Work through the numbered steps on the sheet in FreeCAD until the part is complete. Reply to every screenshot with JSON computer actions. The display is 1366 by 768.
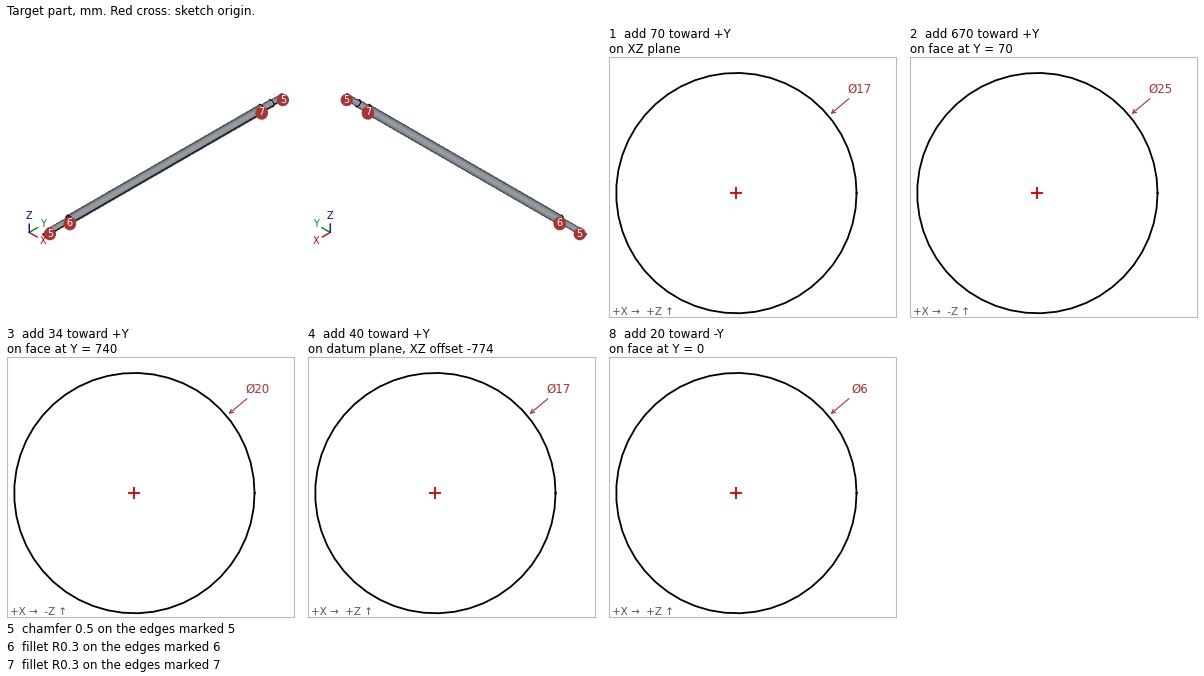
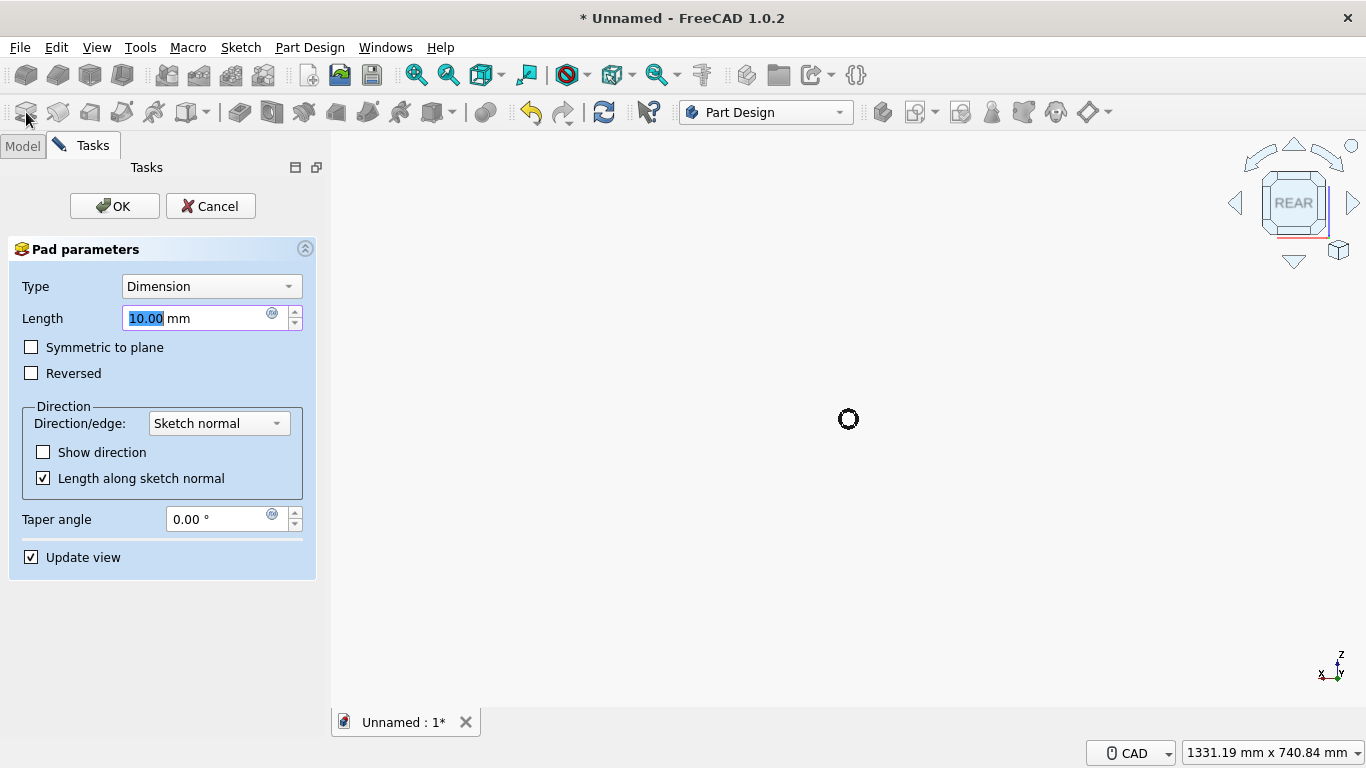
{"action": "type", "text": "34"}
{"action": "key", "text": "Tab"}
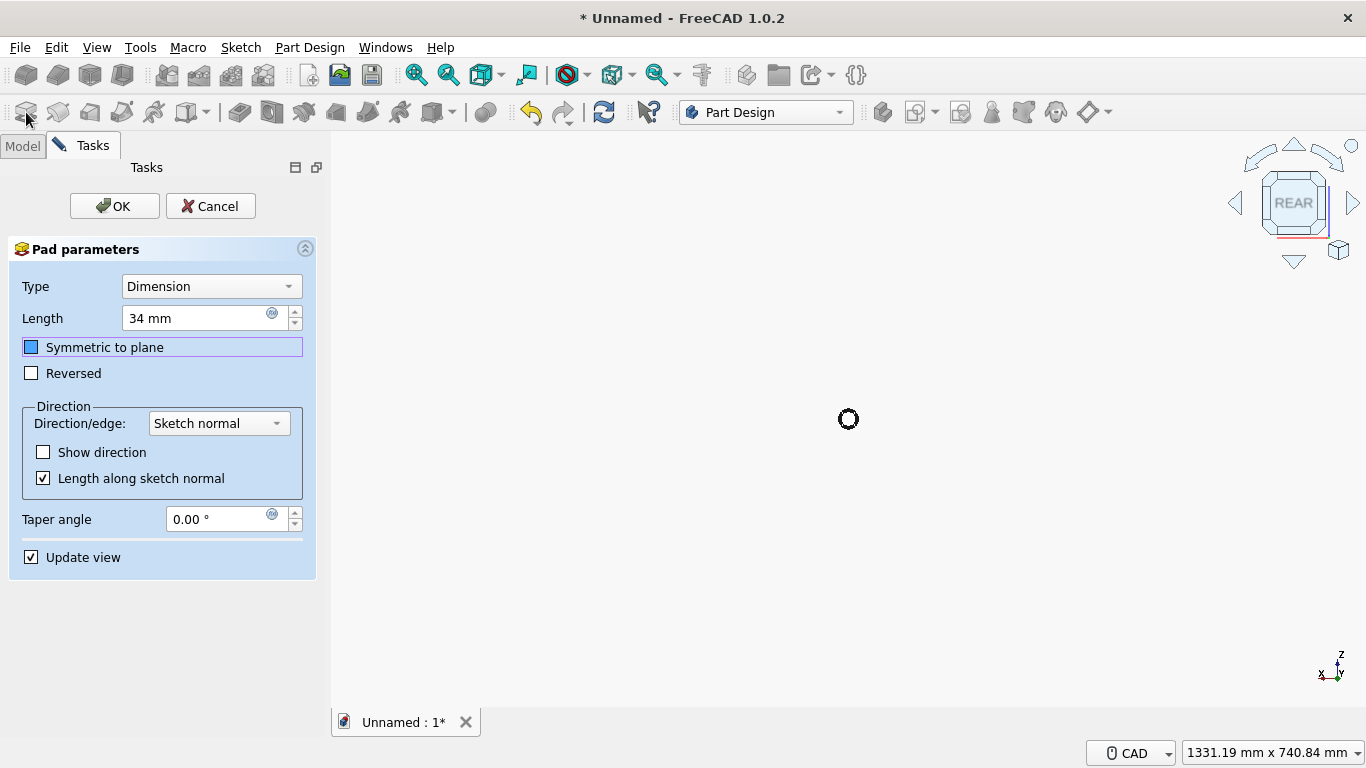
{"action": "left_click", "coordinate": [115, 206]}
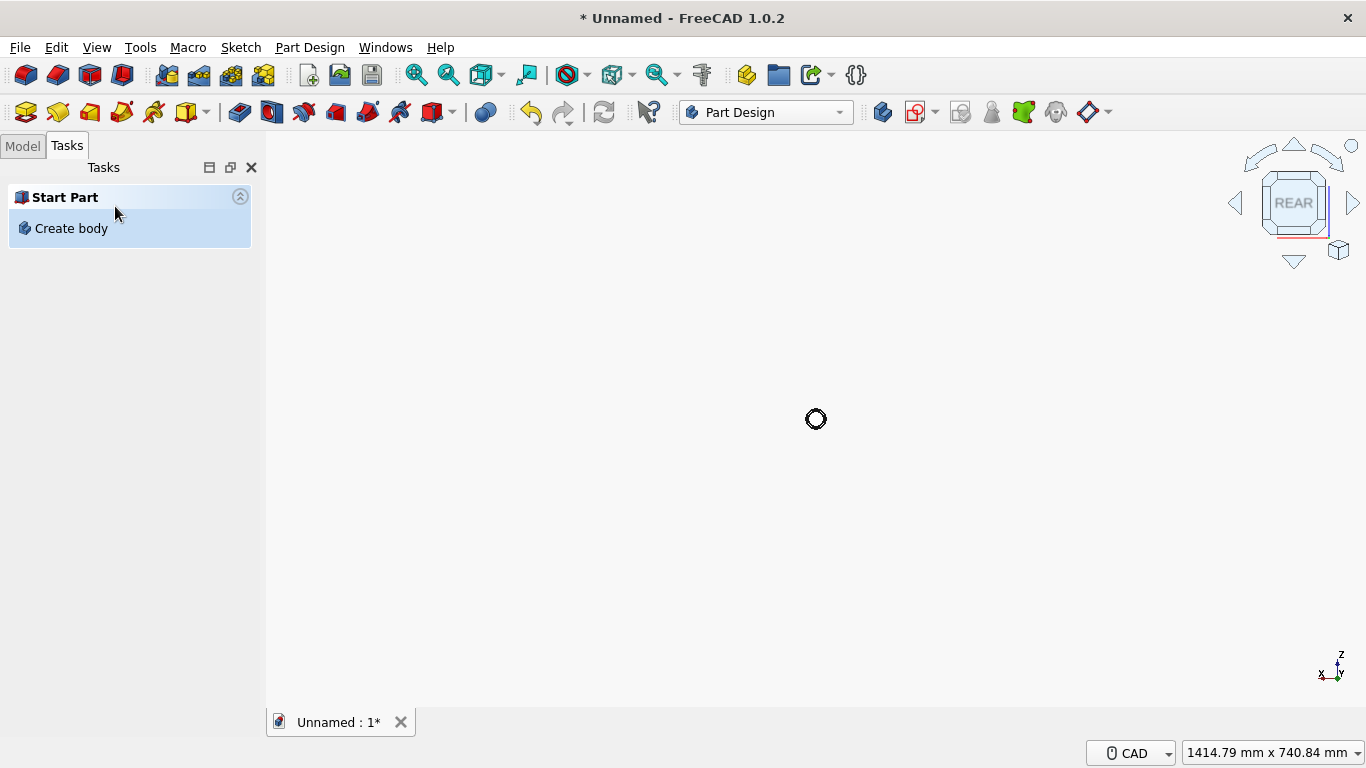
{"action": "left_click", "coordinate": [418, 76]}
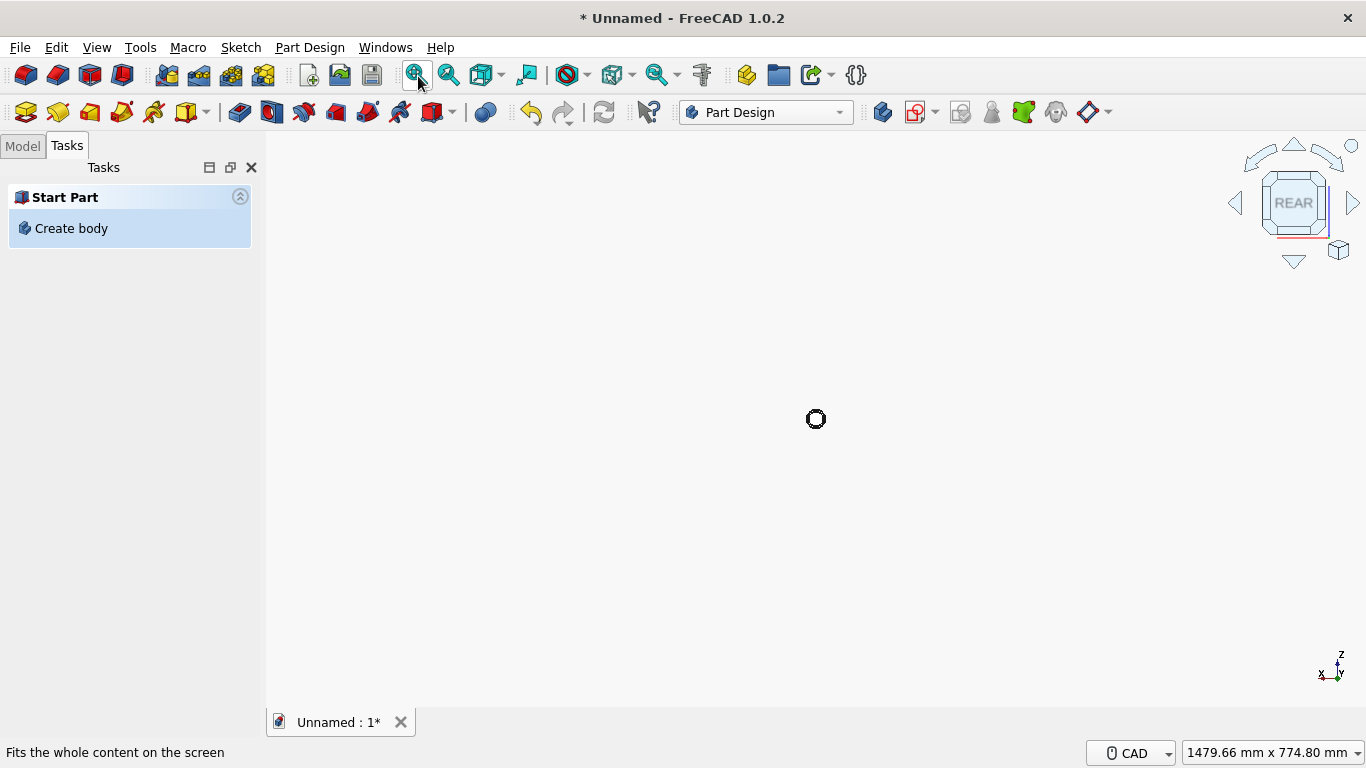
{"action": "key", "text": "5"}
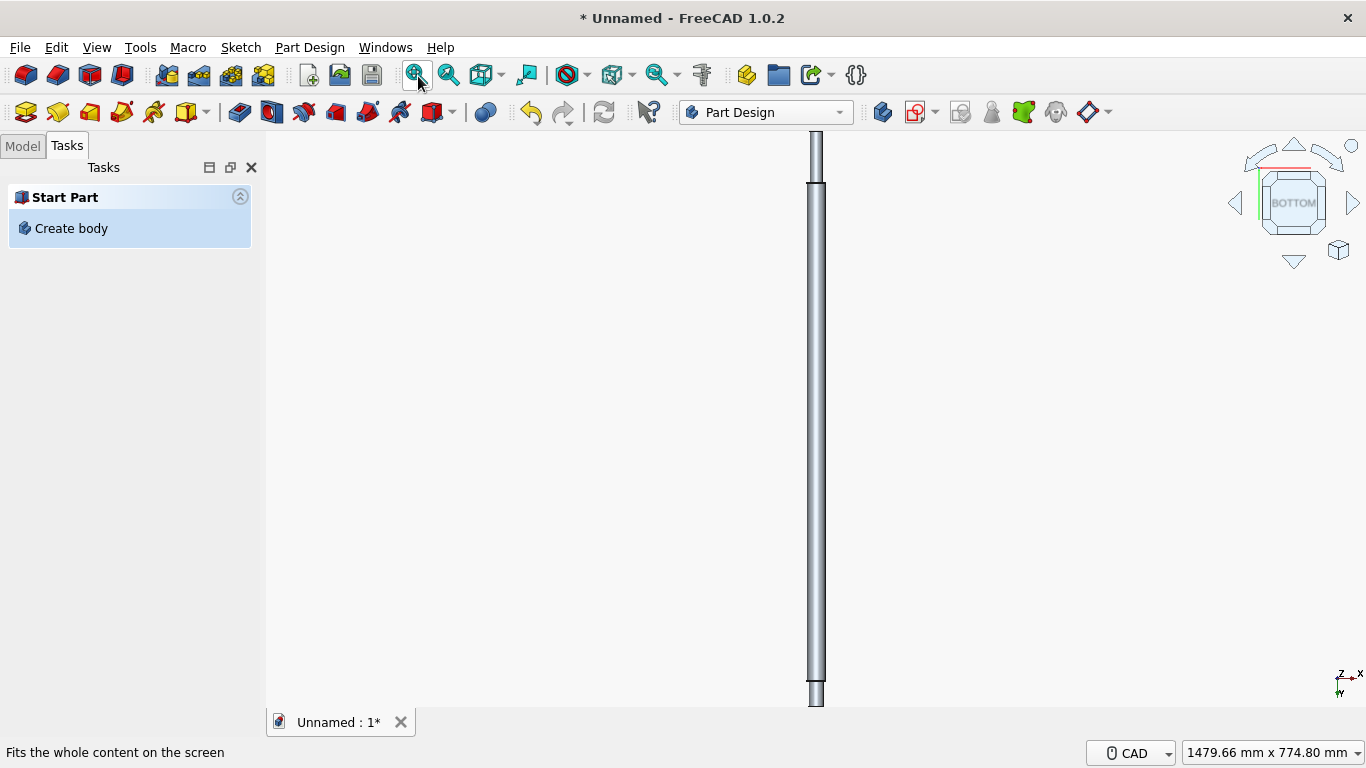
{"action": "left_click", "coordinate": [418, 76]}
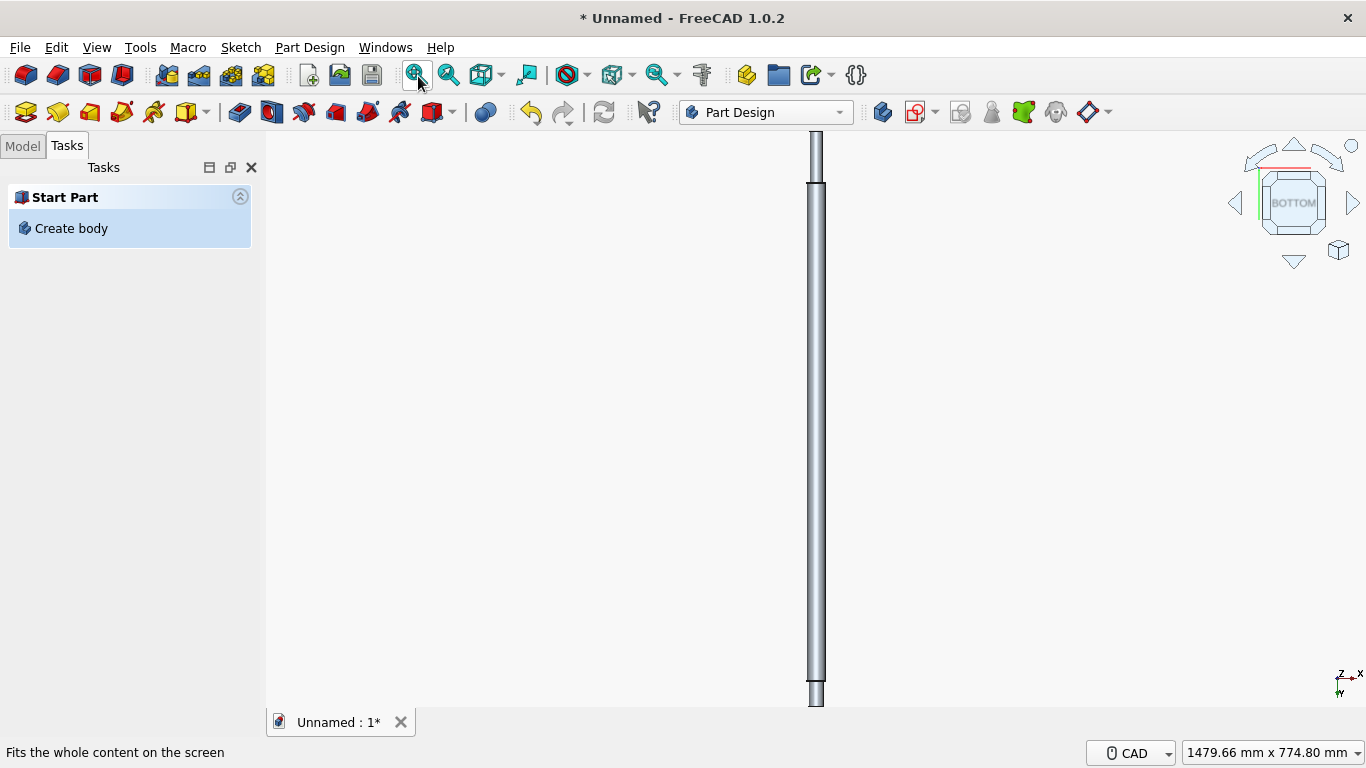
{"action": "key", "text": "4"}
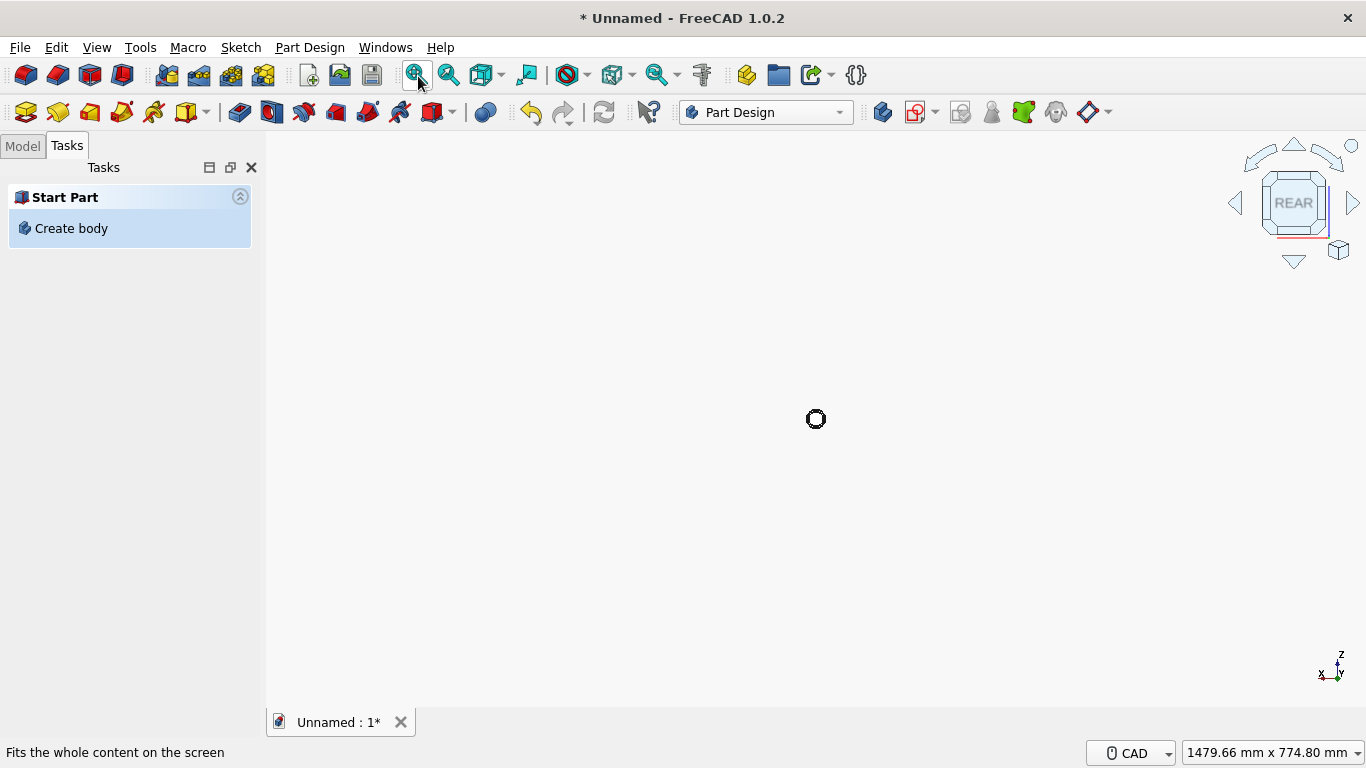
{"action": "left_click", "coordinate": [418, 76]}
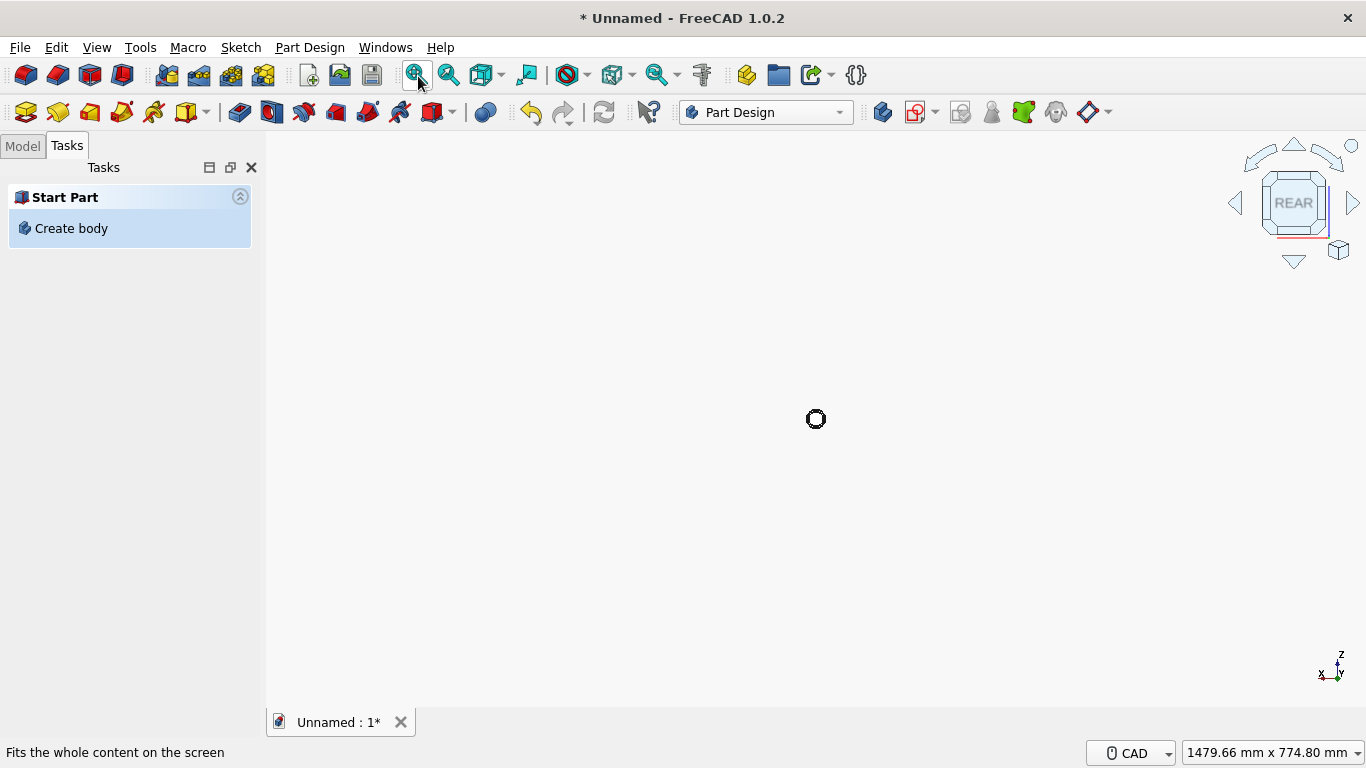
{"action": "key", "text": "3"}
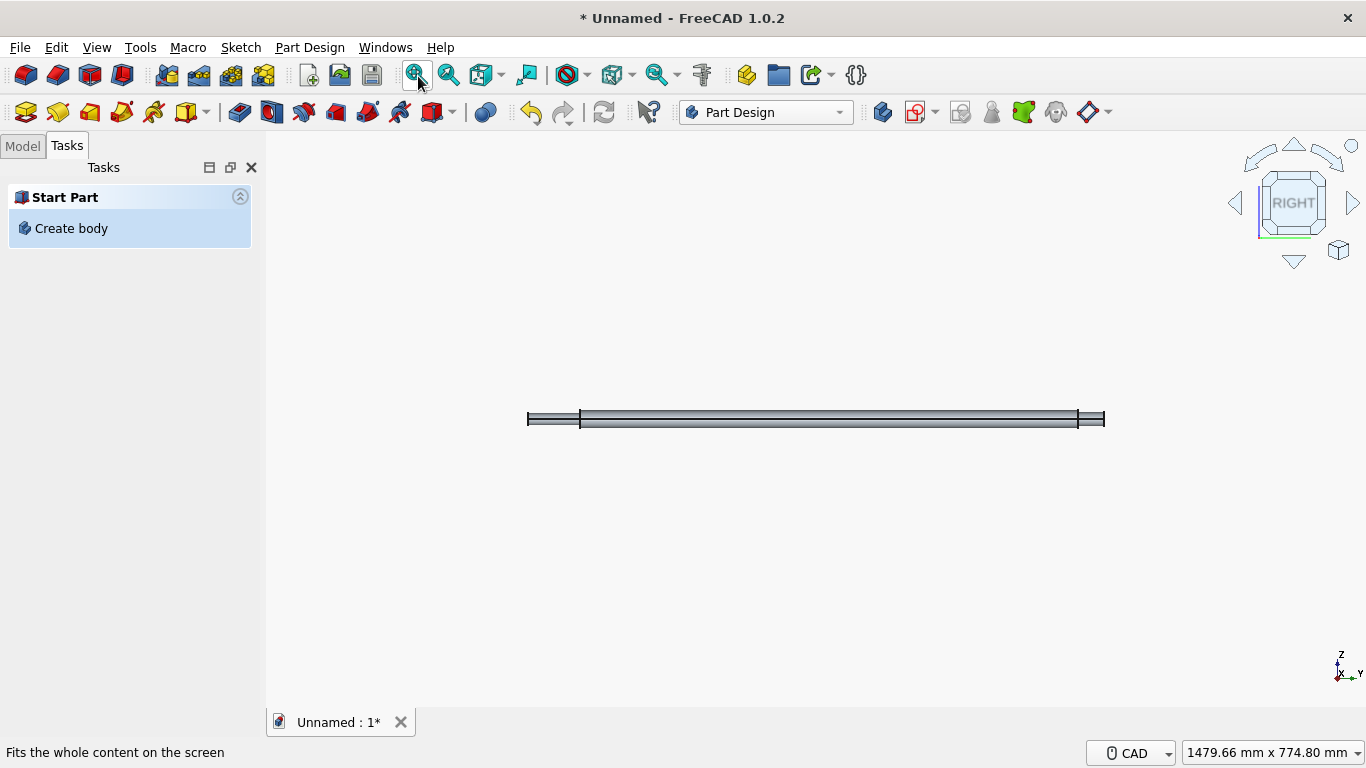
{"action": "left_click", "coordinate": [23, 145]}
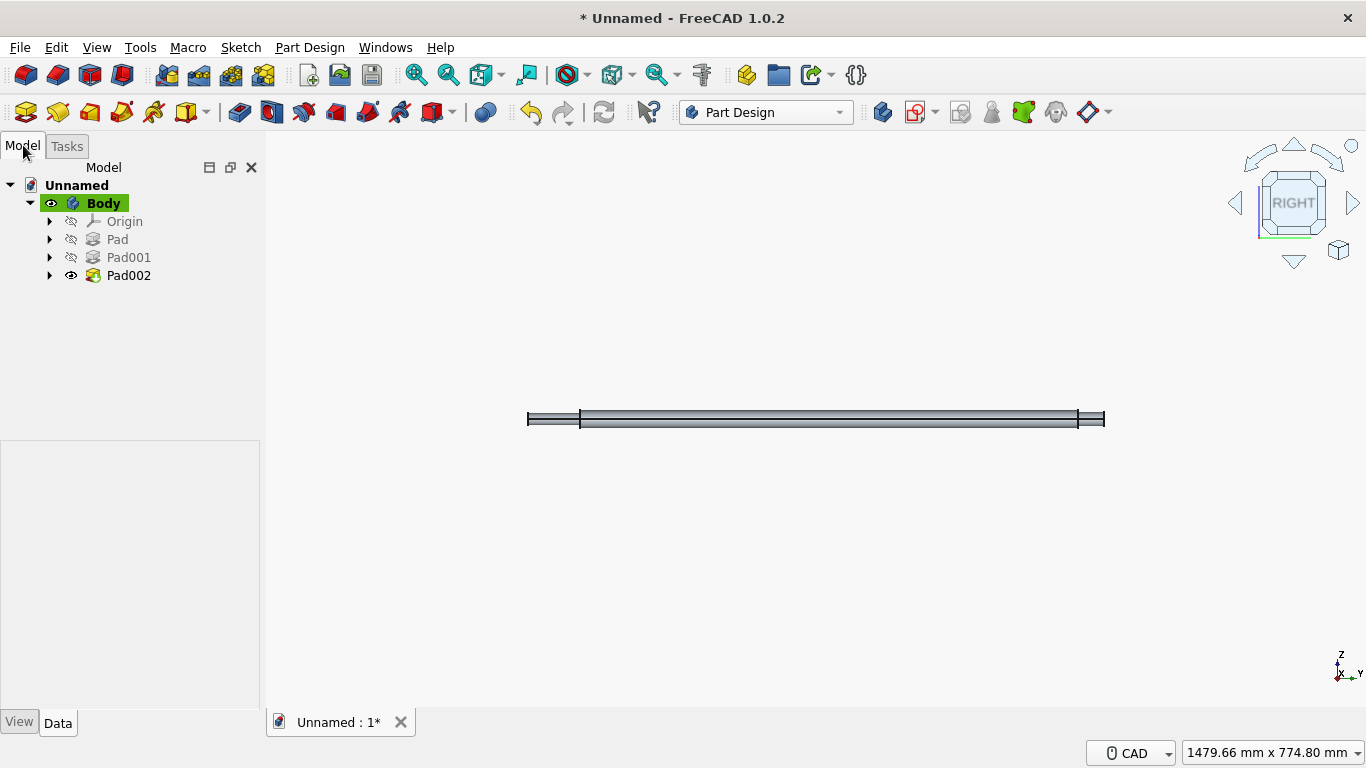
{"action": "left_click", "coordinate": [50, 221]}